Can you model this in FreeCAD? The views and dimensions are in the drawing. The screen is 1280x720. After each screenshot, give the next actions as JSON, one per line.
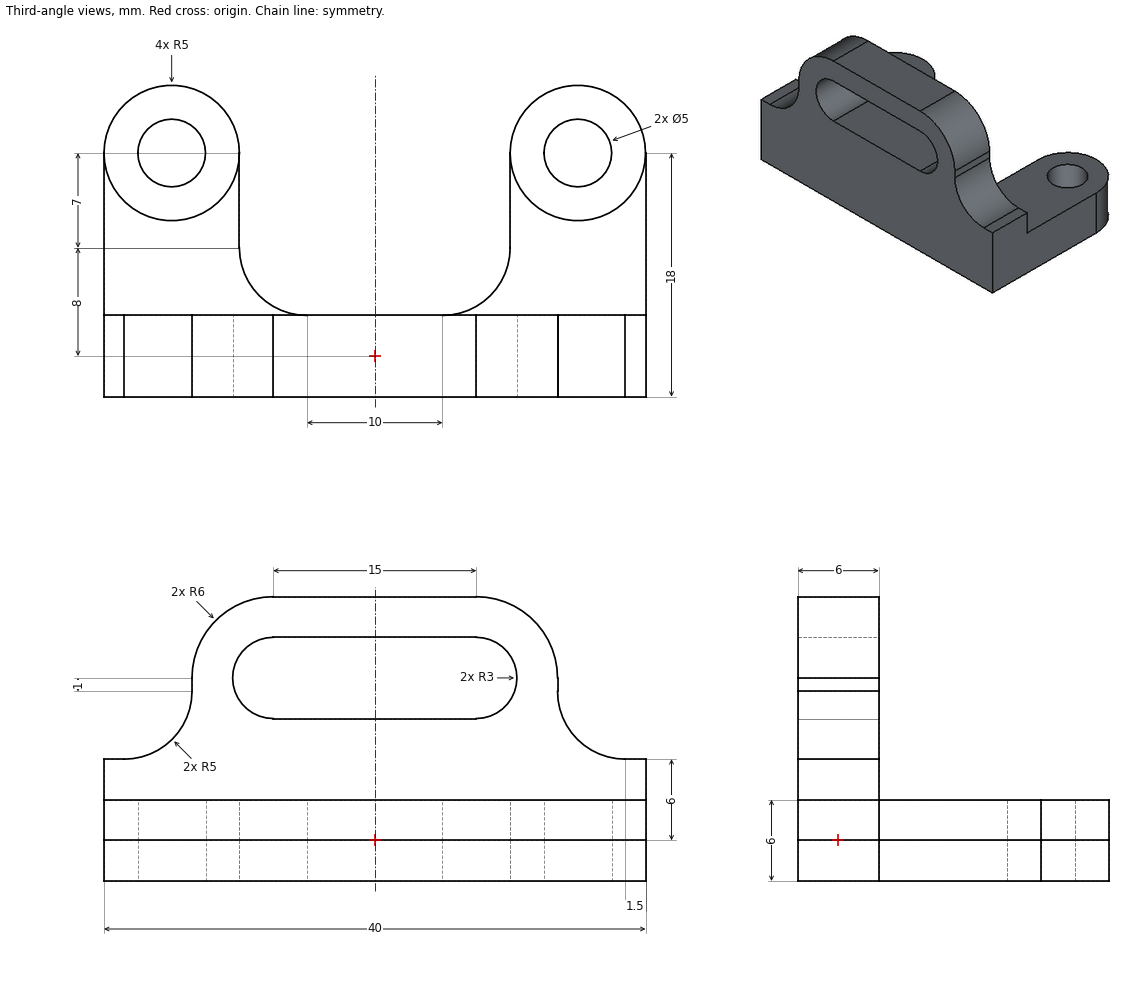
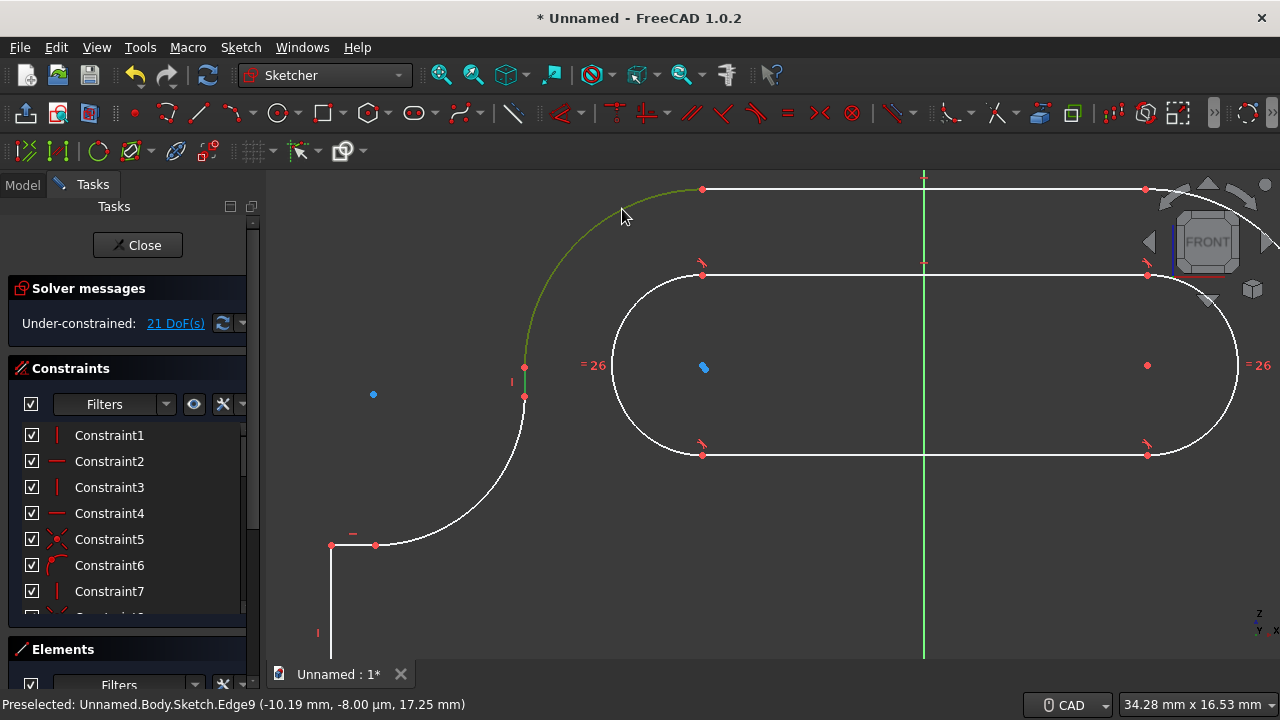
{"action": "left_click", "coordinate": [756, 114]}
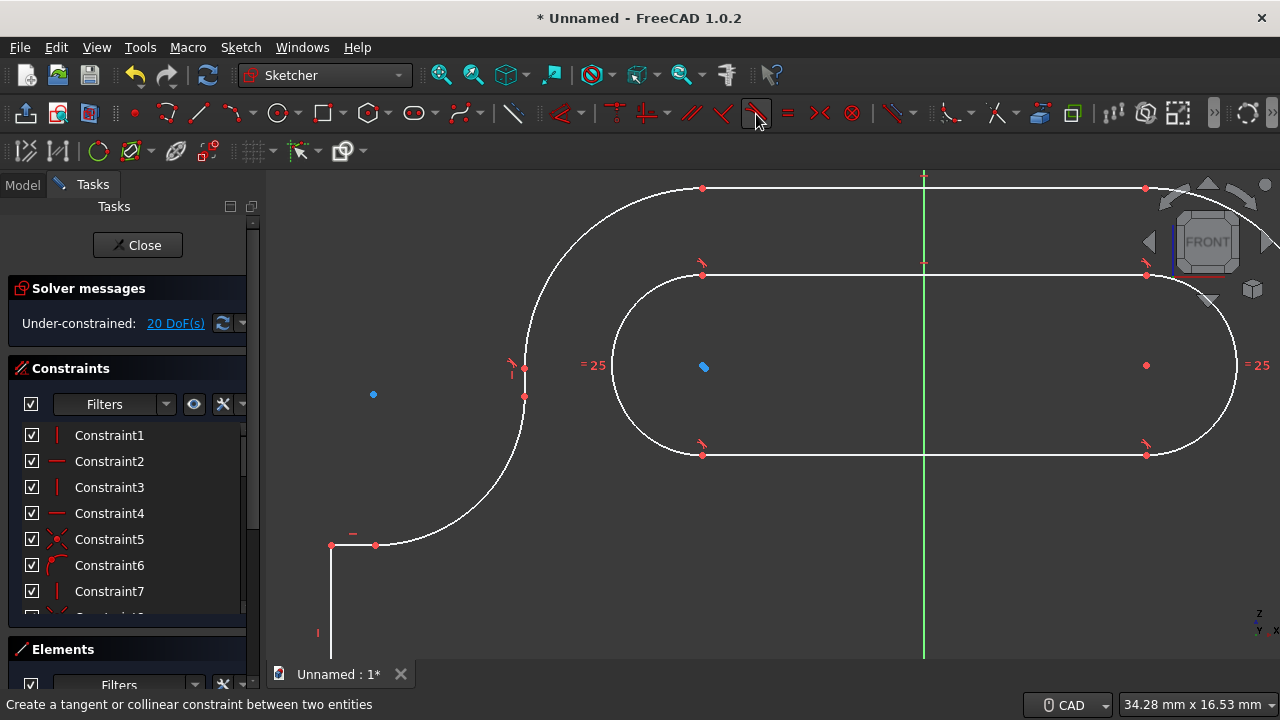
{"action": "scroll", "coordinate": [525, 385], "scroll_direction": "up", "scroll_amount": 2}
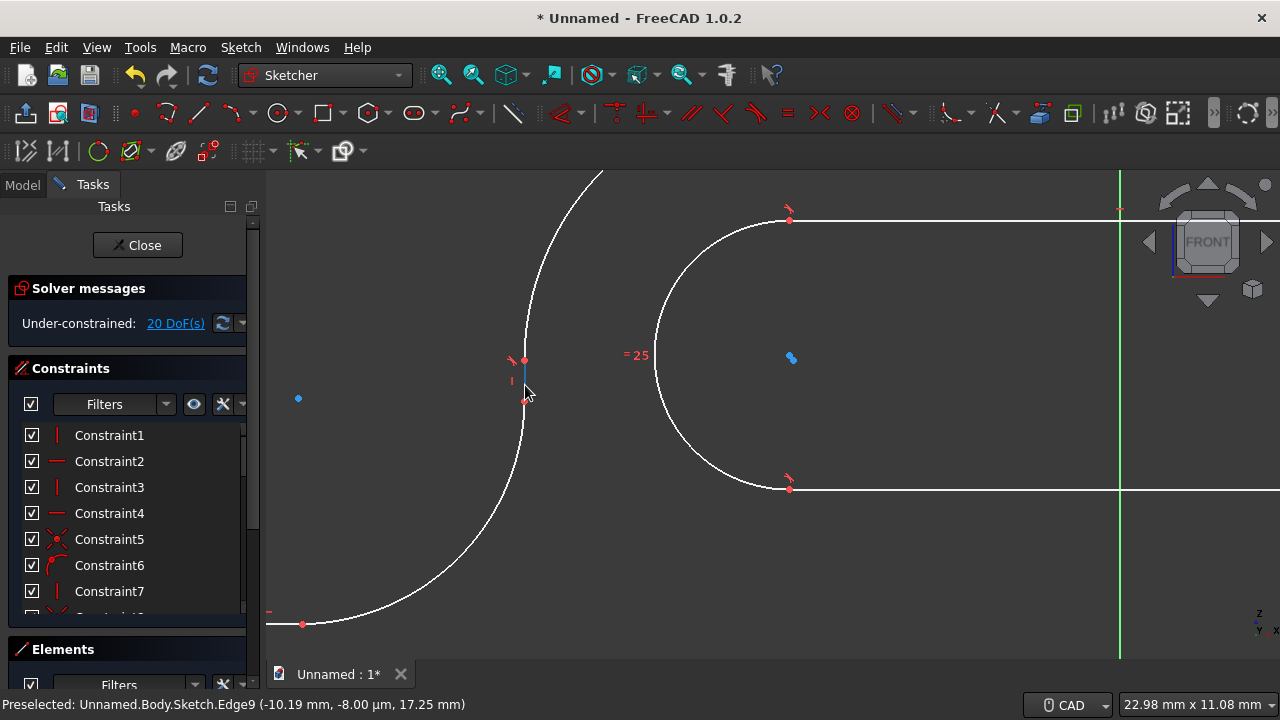
{"action": "left_click", "coordinate": [525, 385]}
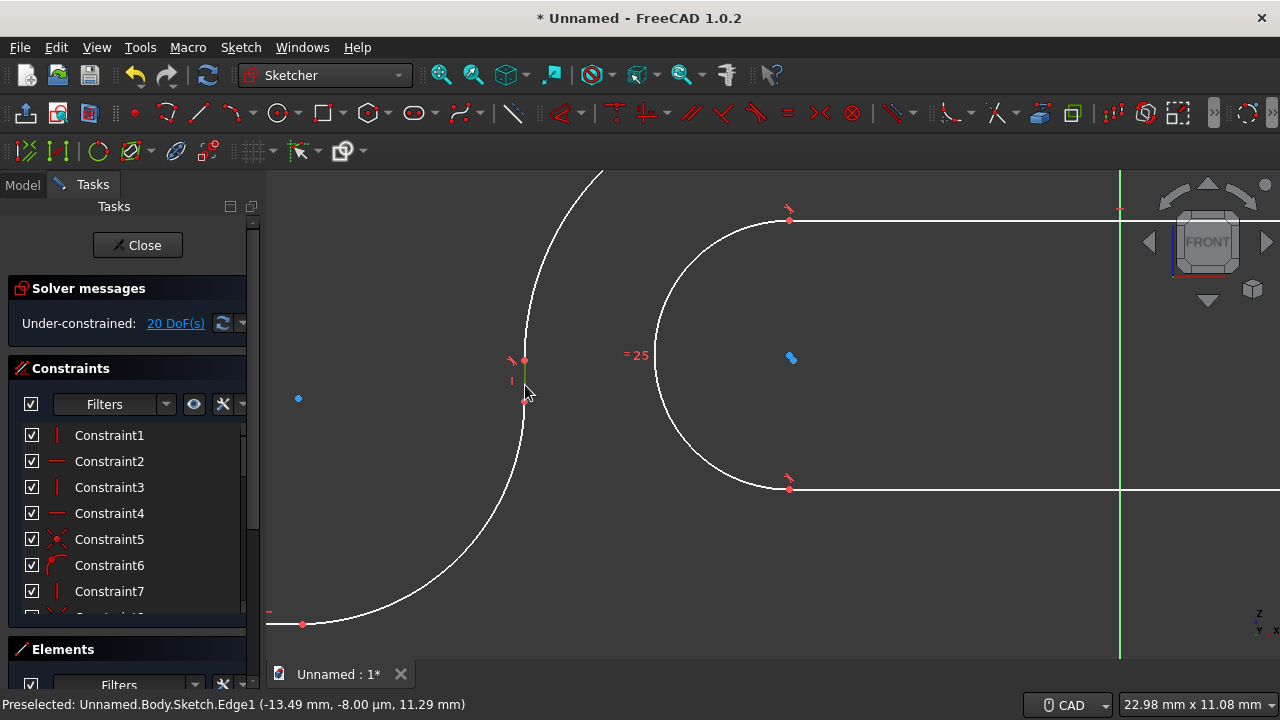
{"action": "left_click", "coordinate": [402, 599]}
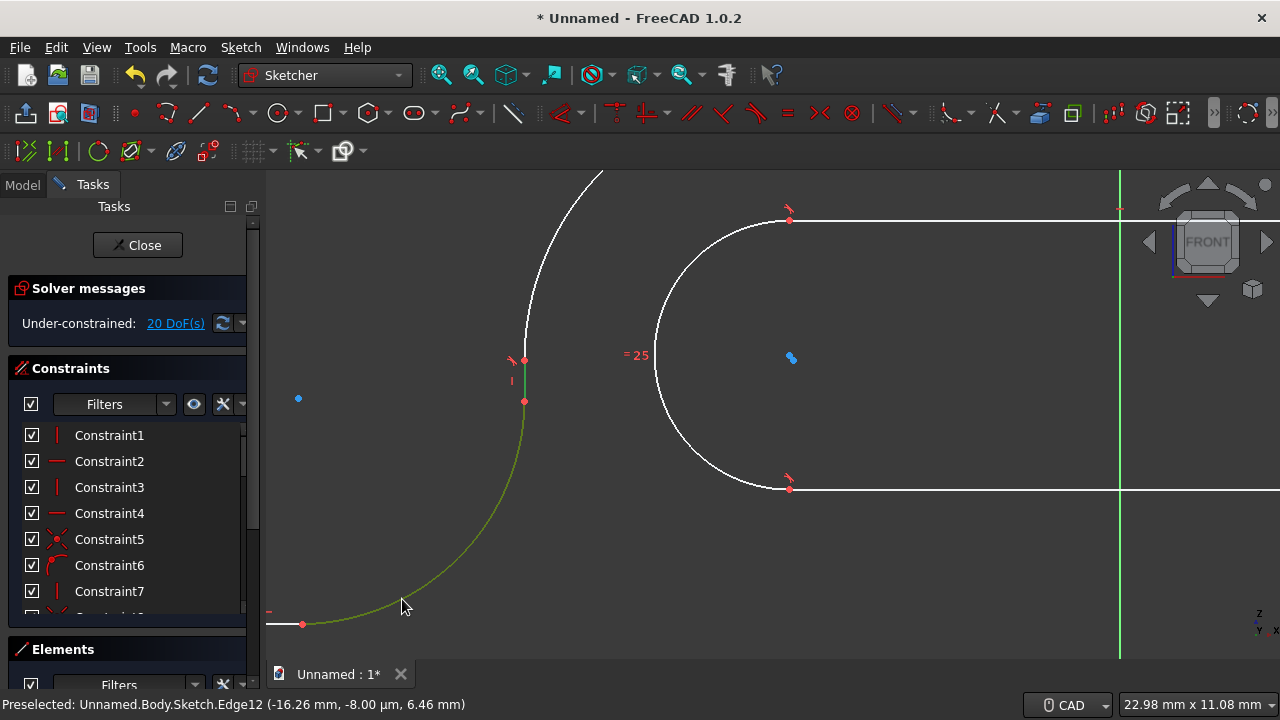
{"action": "left_click", "coordinate": [756, 114]}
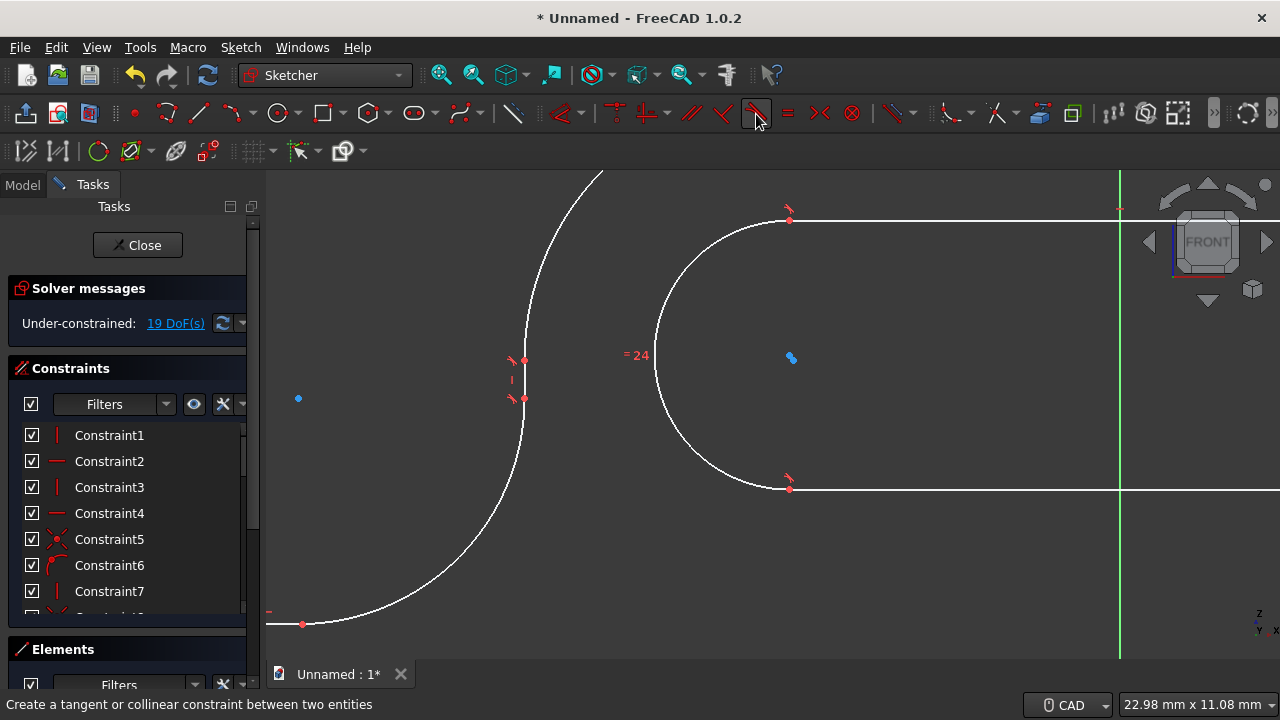
{"action": "scroll", "coordinate": [525, 383], "scroll_direction": "down", "scroll_amount": 6}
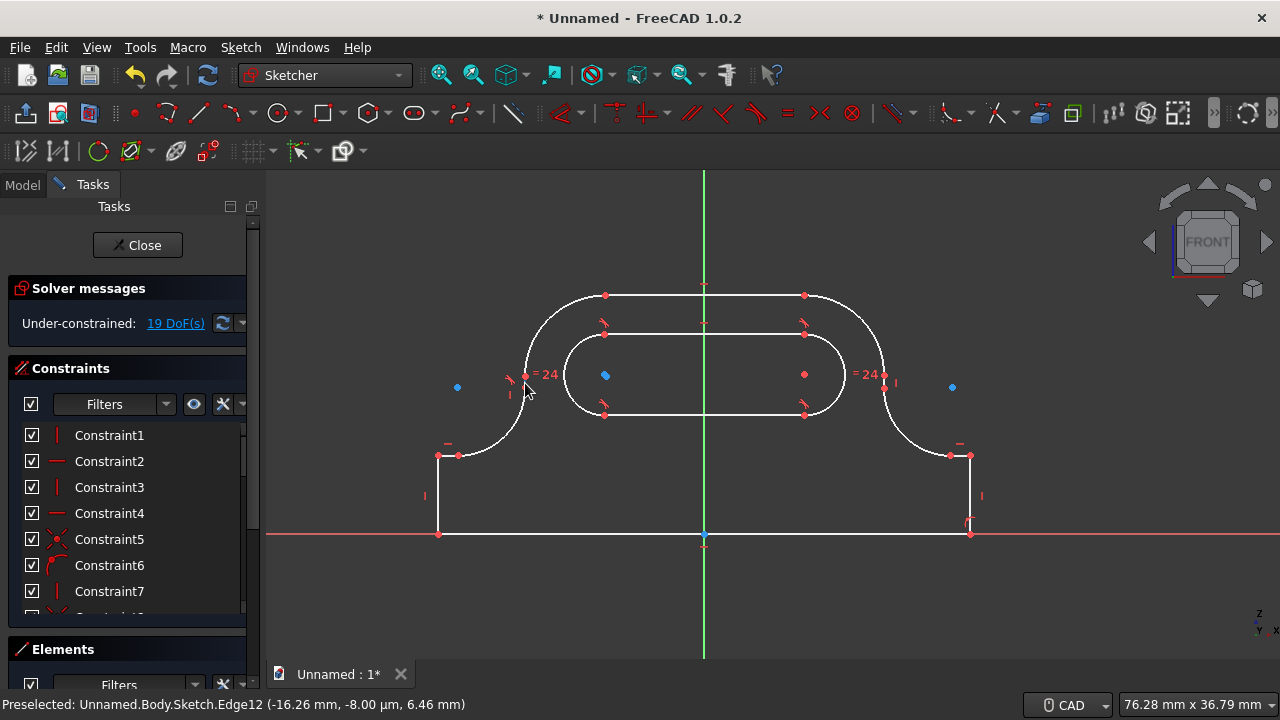
{"action": "left_click", "coordinate": [665, 295]}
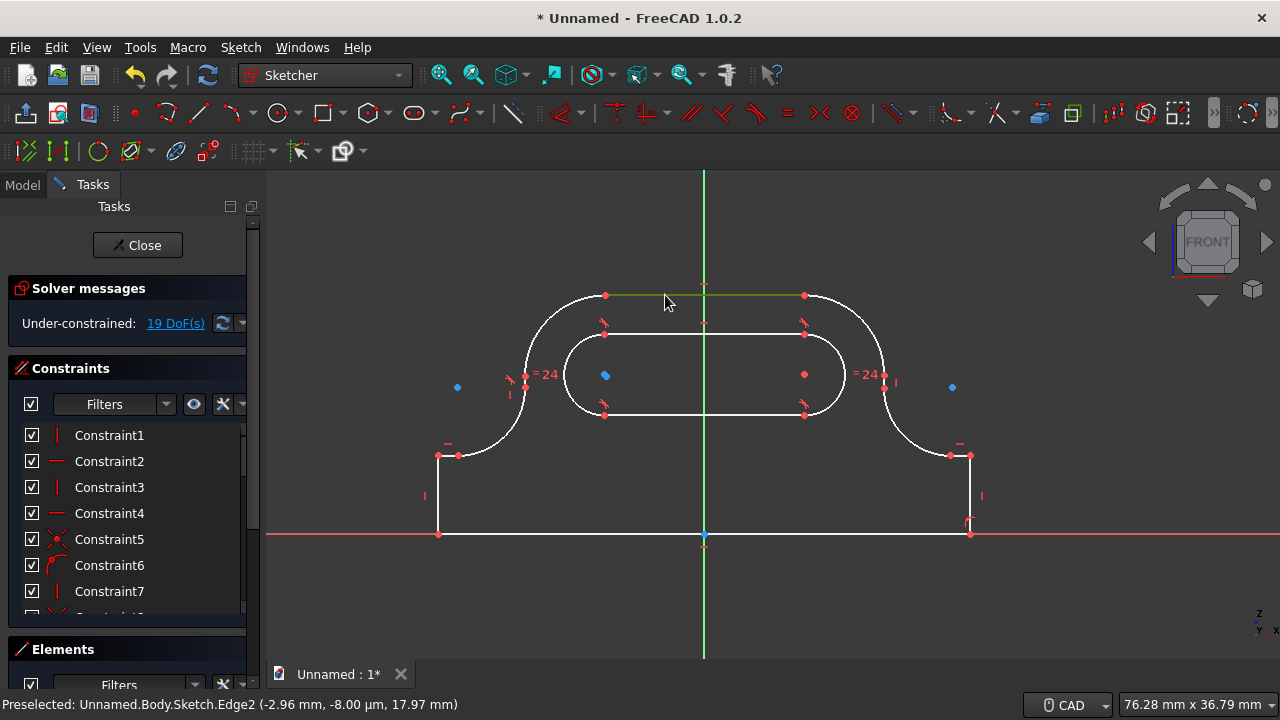
{"action": "left_click", "coordinate": [569, 305]}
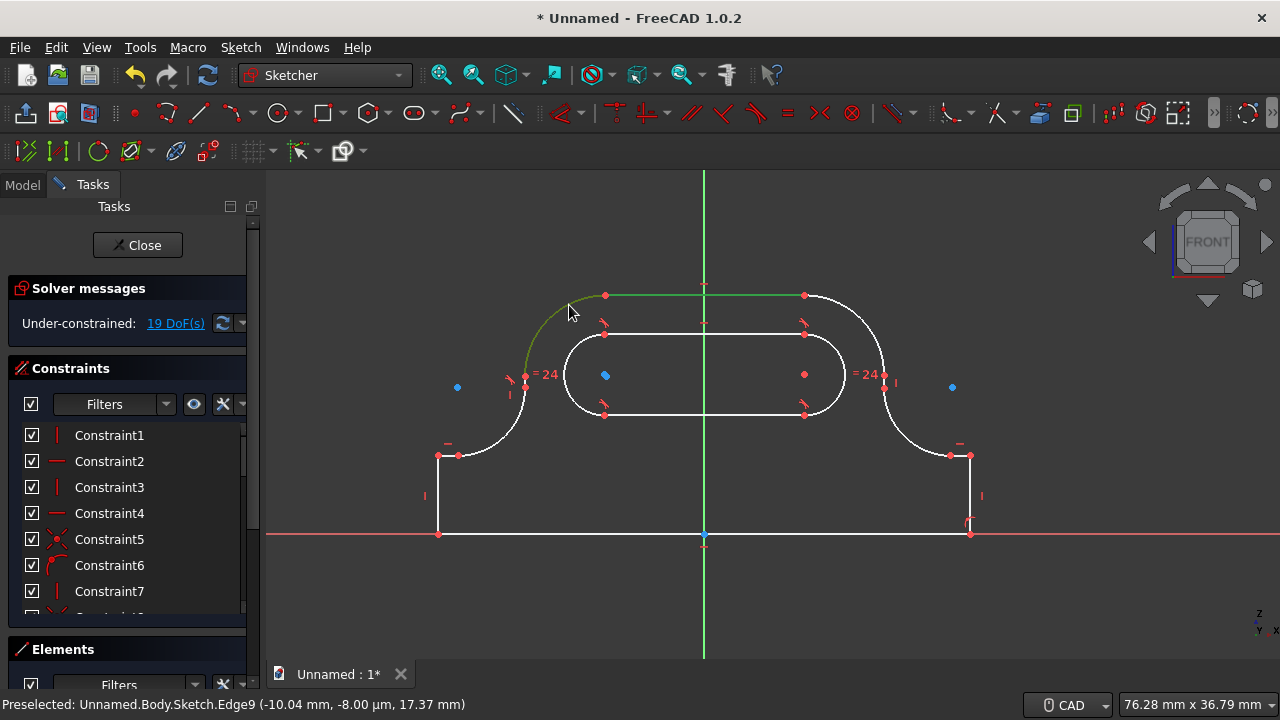
{"action": "left_click", "coordinate": [756, 114]}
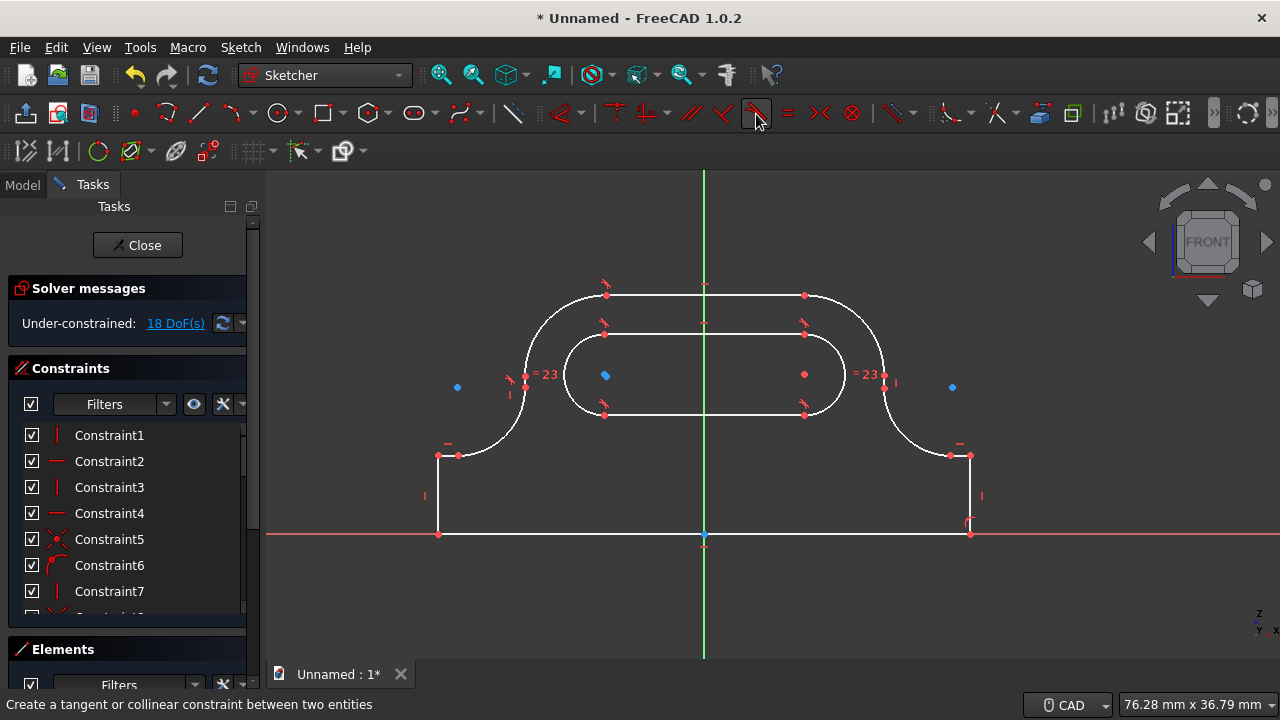
{"action": "left_click", "coordinate": [665, 295]}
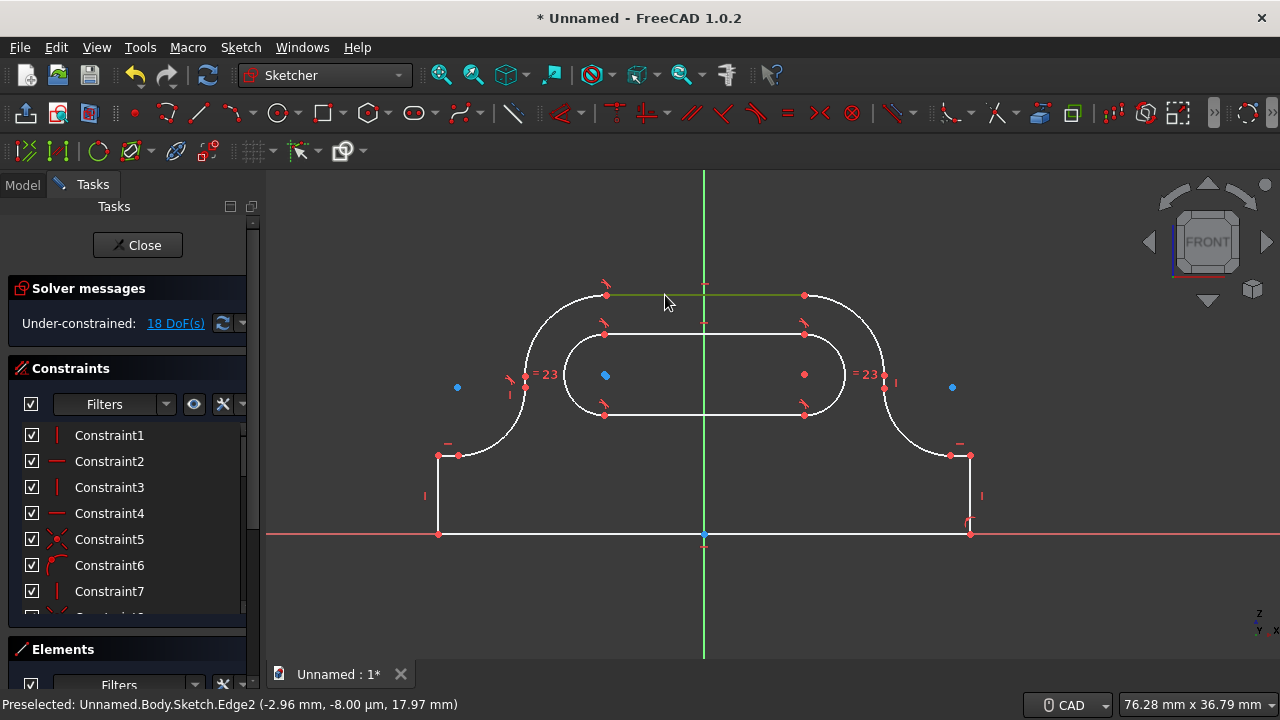
{"action": "left_click", "coordinate": [876, 339]}